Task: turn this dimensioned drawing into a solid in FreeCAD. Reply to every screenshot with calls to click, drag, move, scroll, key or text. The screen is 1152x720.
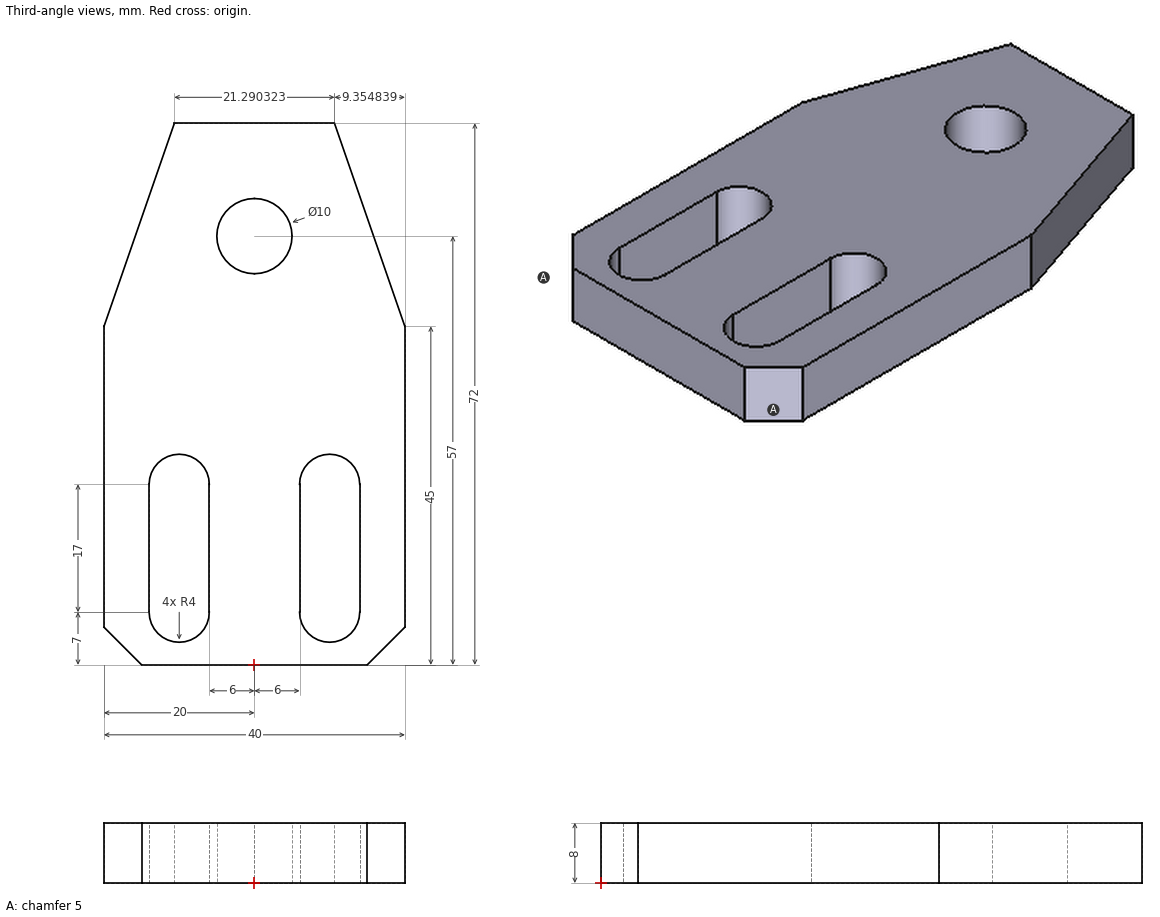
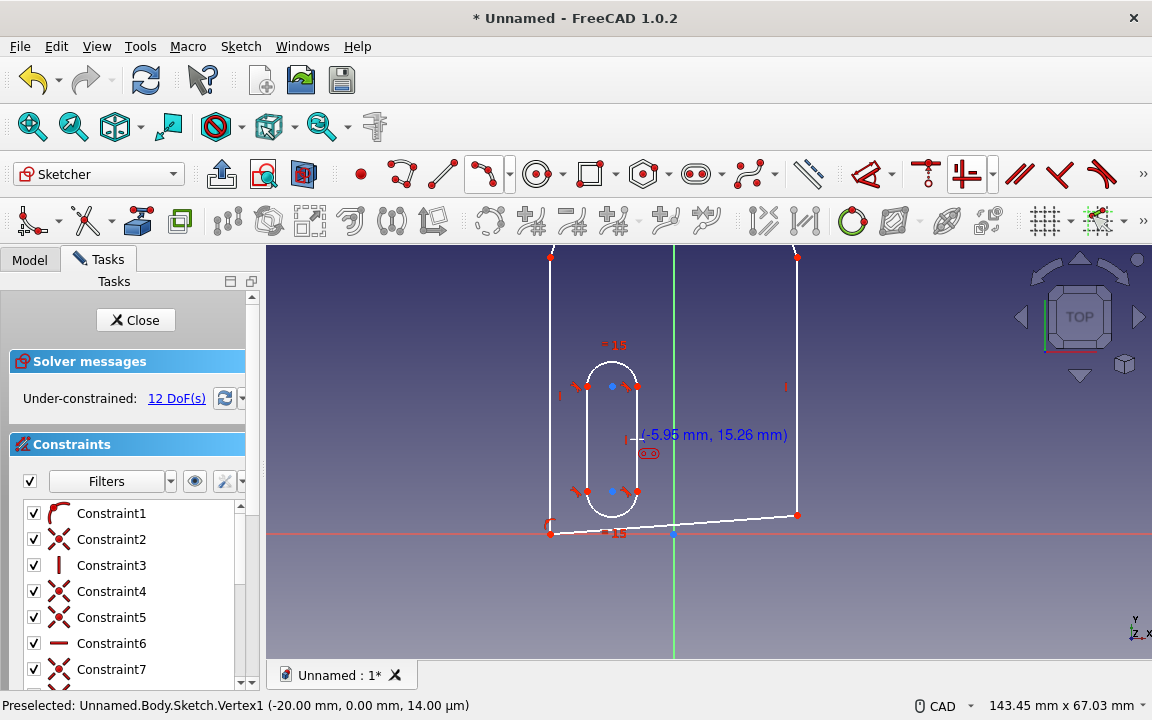
click(736, 491)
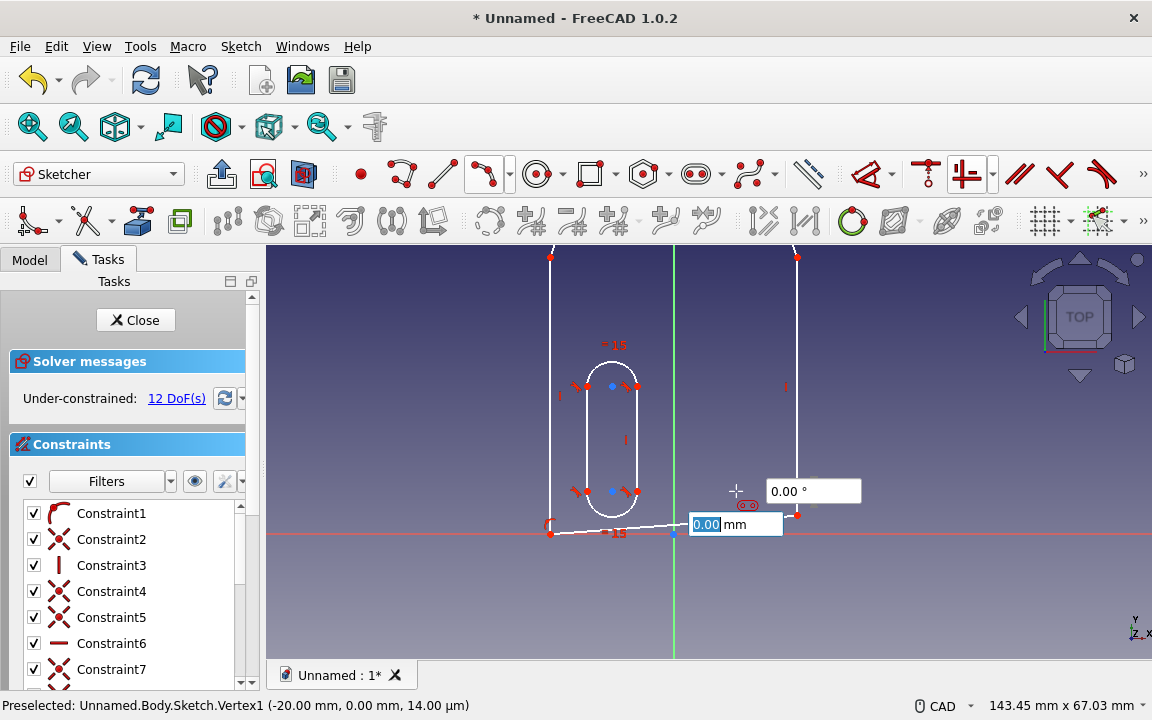
click(736, 386)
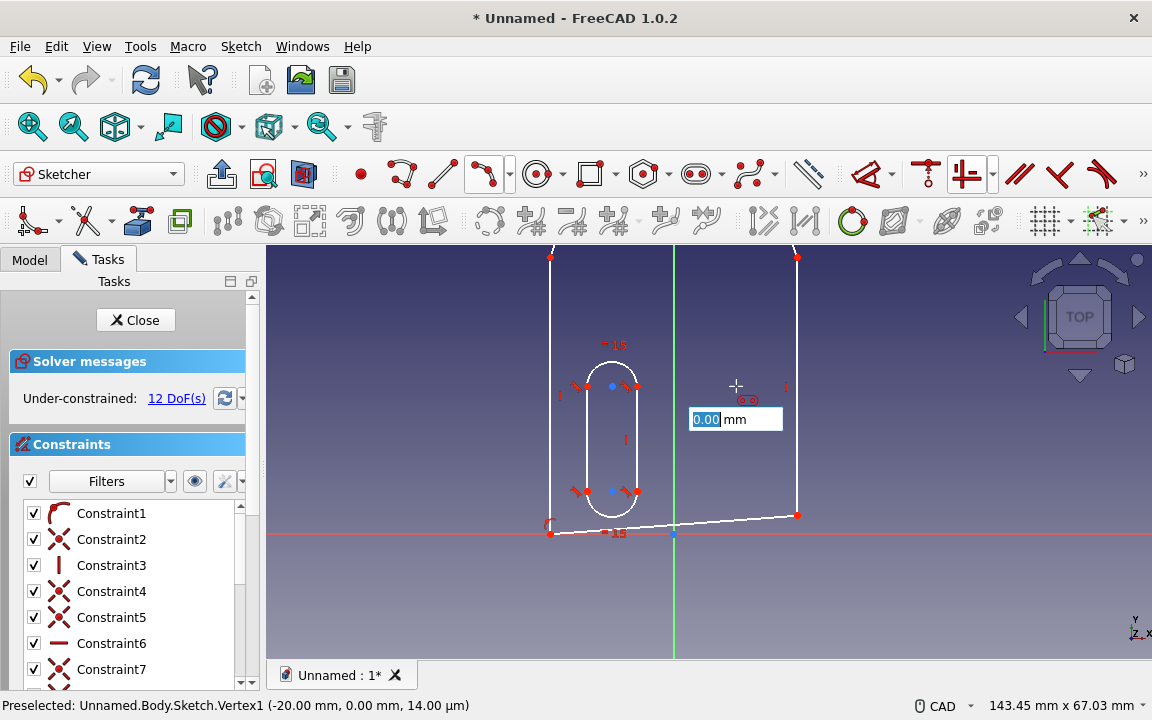
click(711, 439)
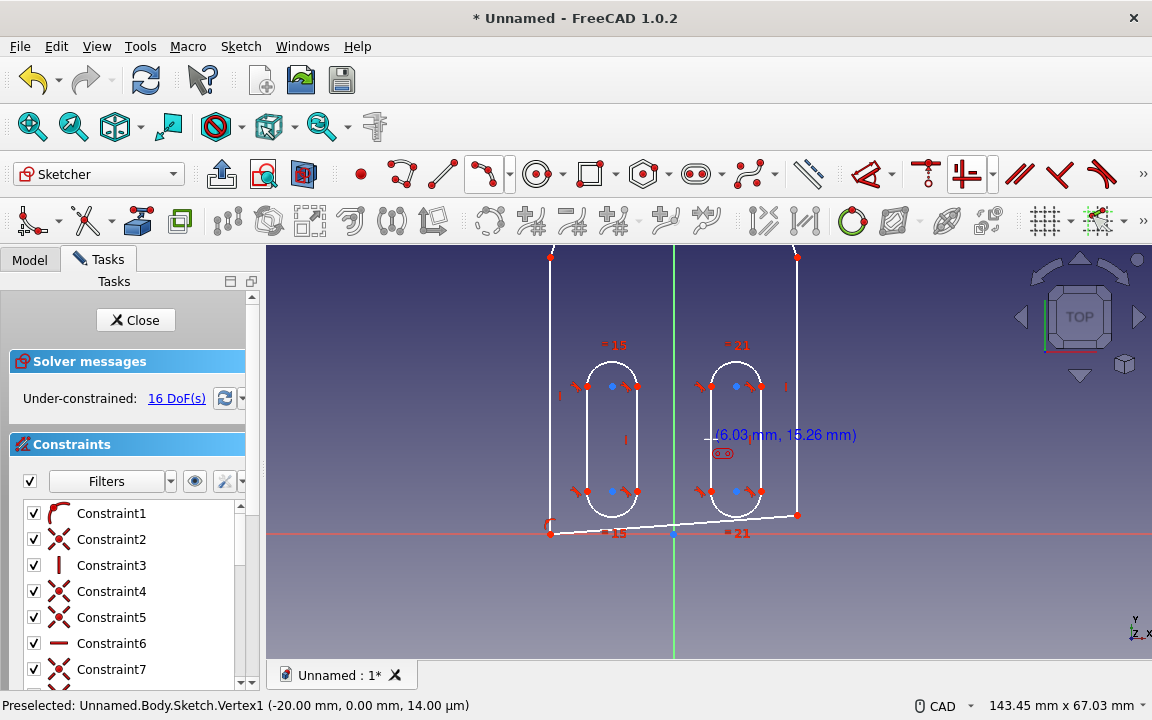
click(536, 174)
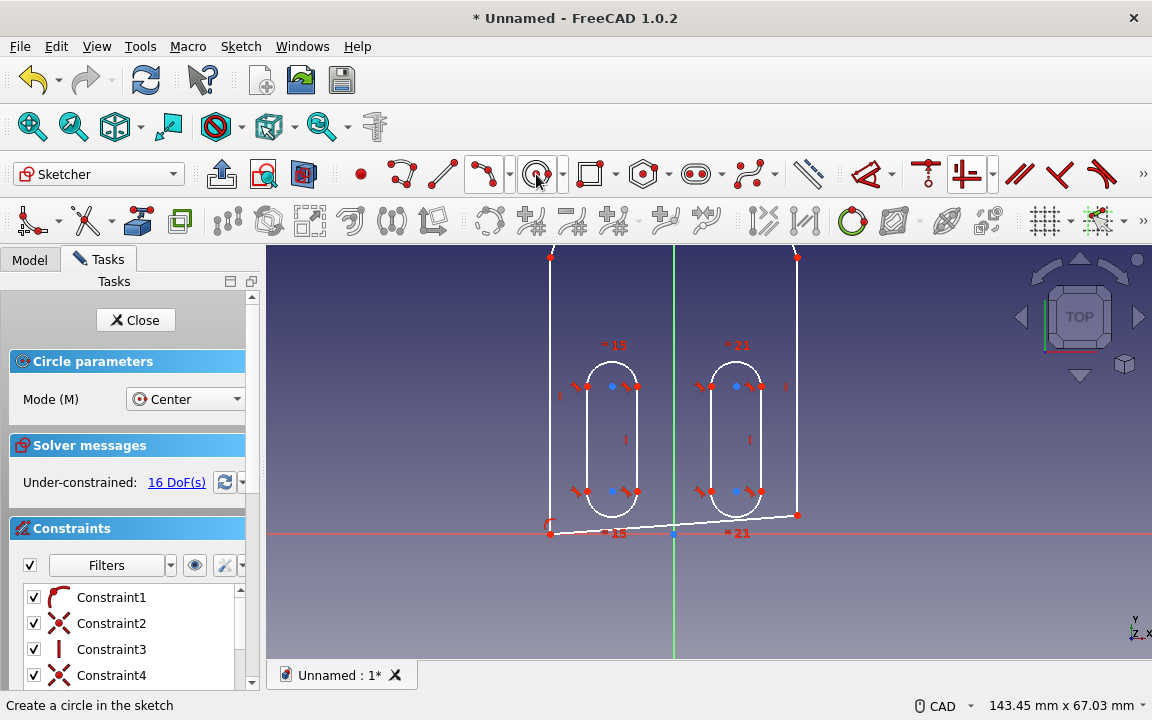
scroll(600, 622, down, 3)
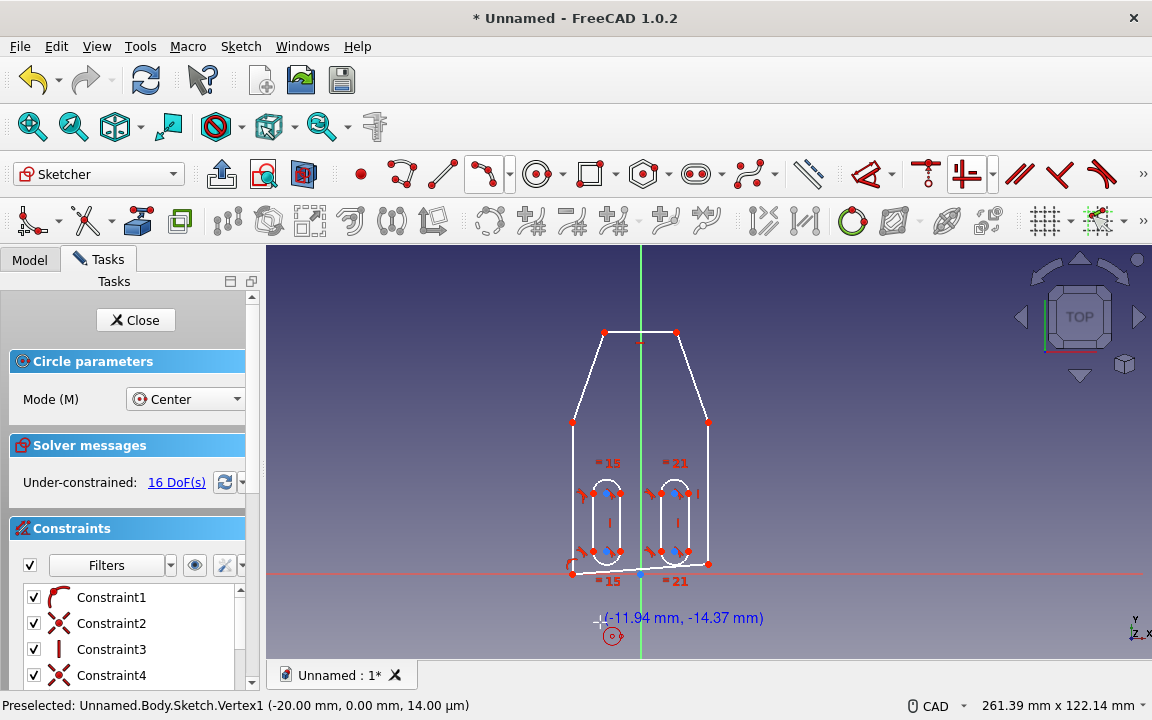
scroll(641, 381, up, 2)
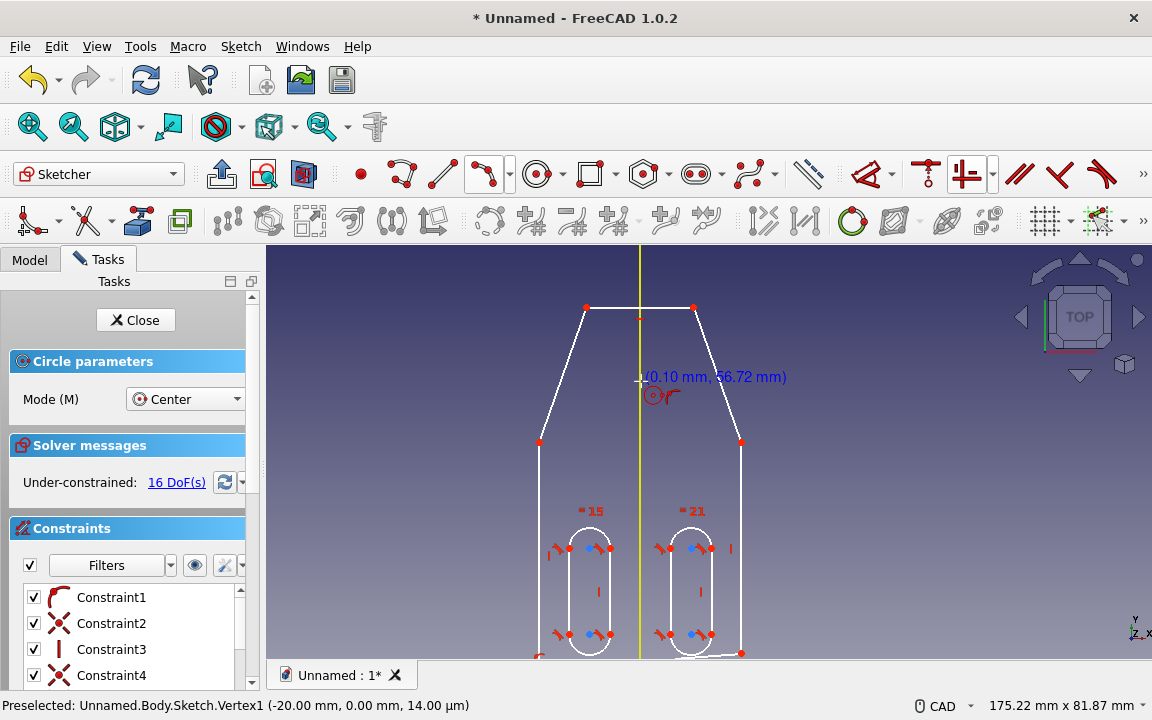
click(640, 381)
click(658, 363)
key(Escape)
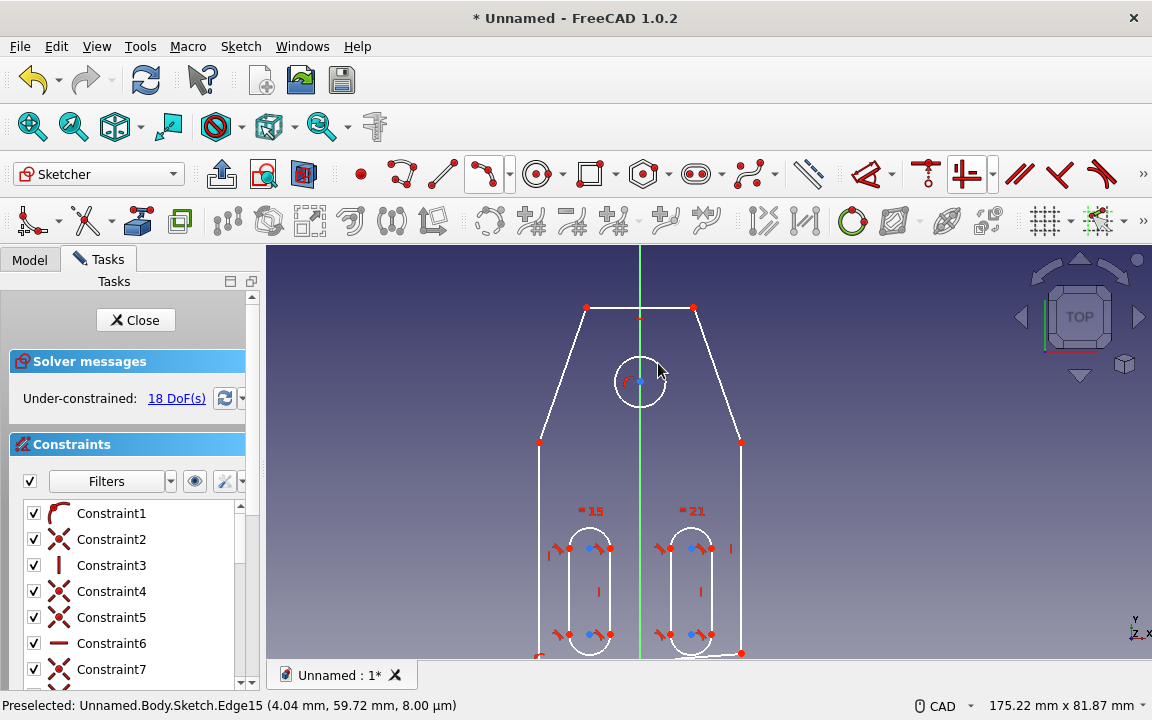
scroll(641, 381, down, 2)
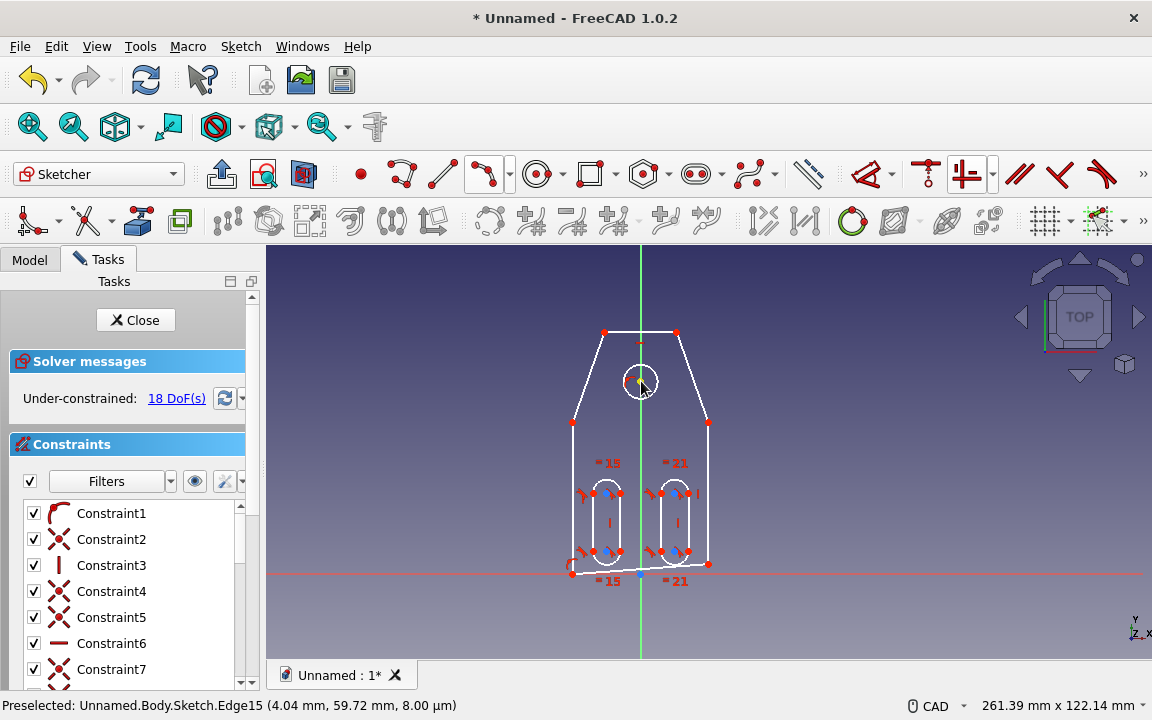
scroll(654, 568, up, 5)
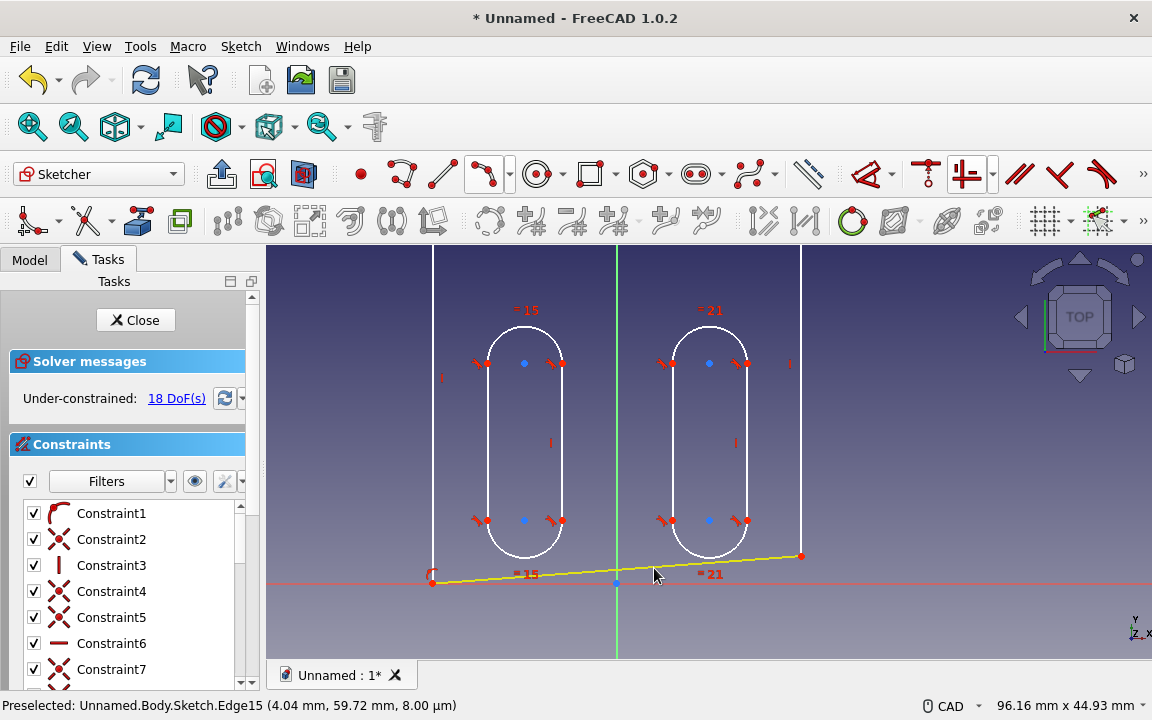
click(654, 567)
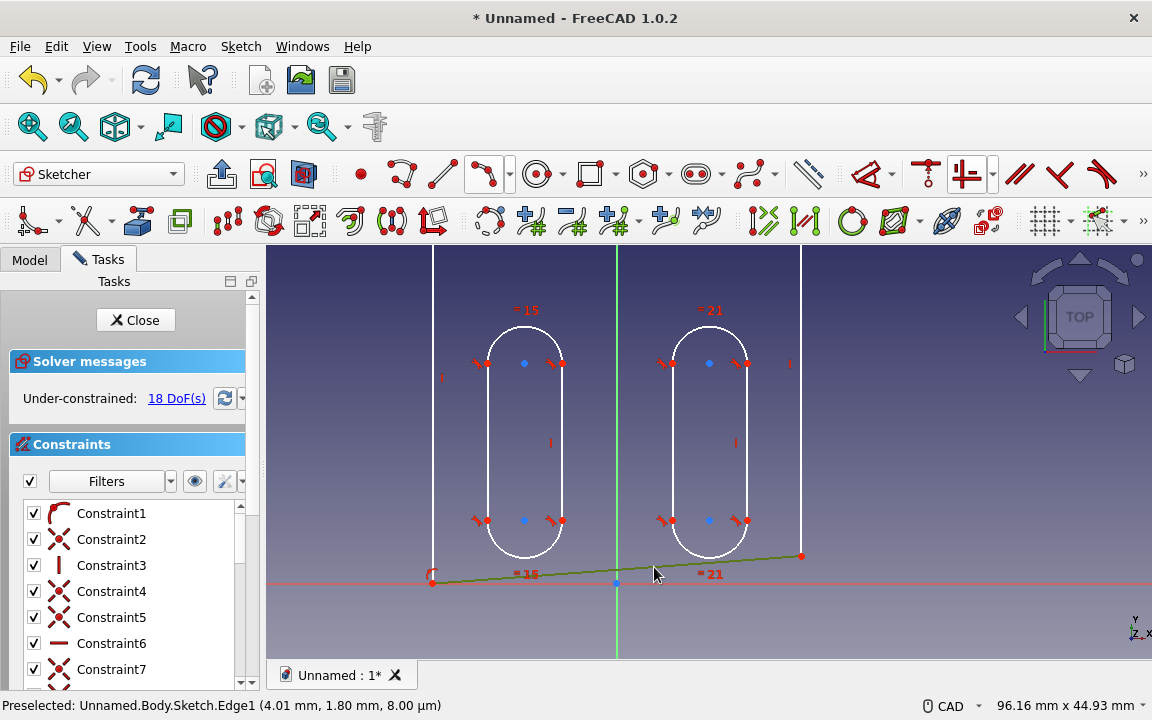
click(992, 174)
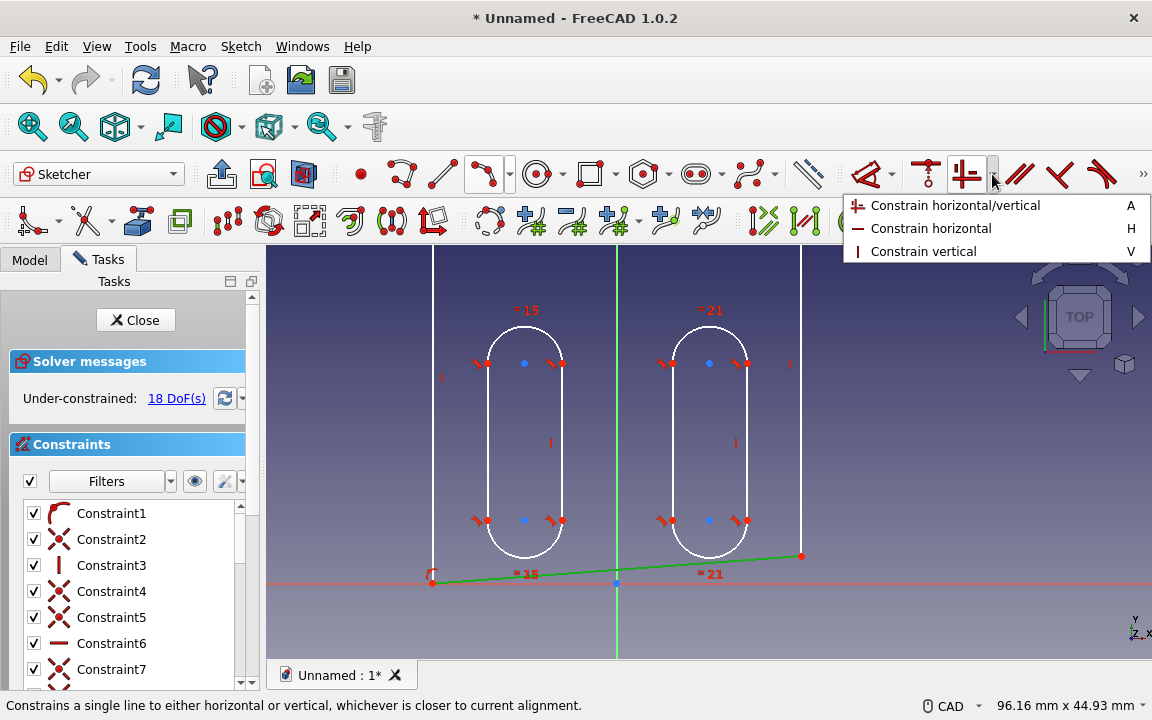
click(997, 228)